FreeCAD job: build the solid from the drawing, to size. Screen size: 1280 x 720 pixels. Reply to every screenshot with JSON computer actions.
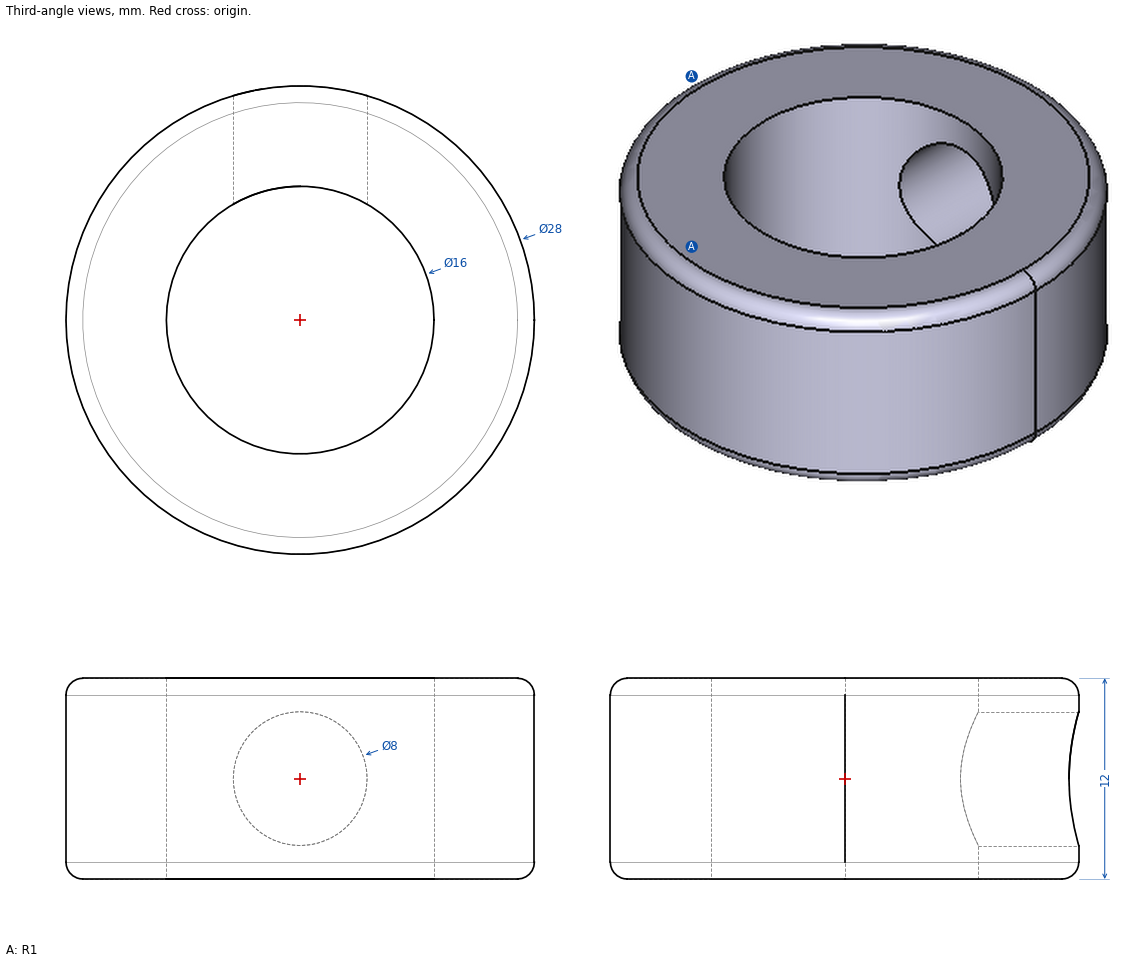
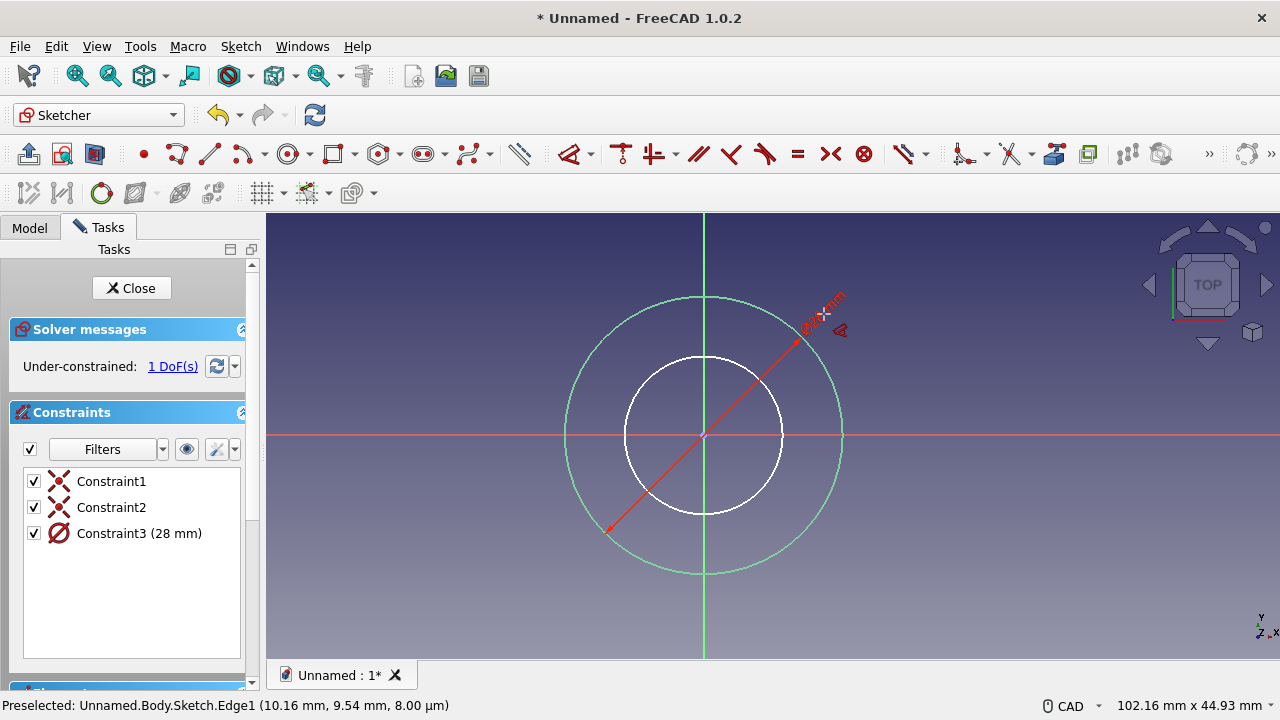
{"action": "left_click", "coordinate": [759, 379]}
{"action": "left_click", "coordinate": [781, 356]}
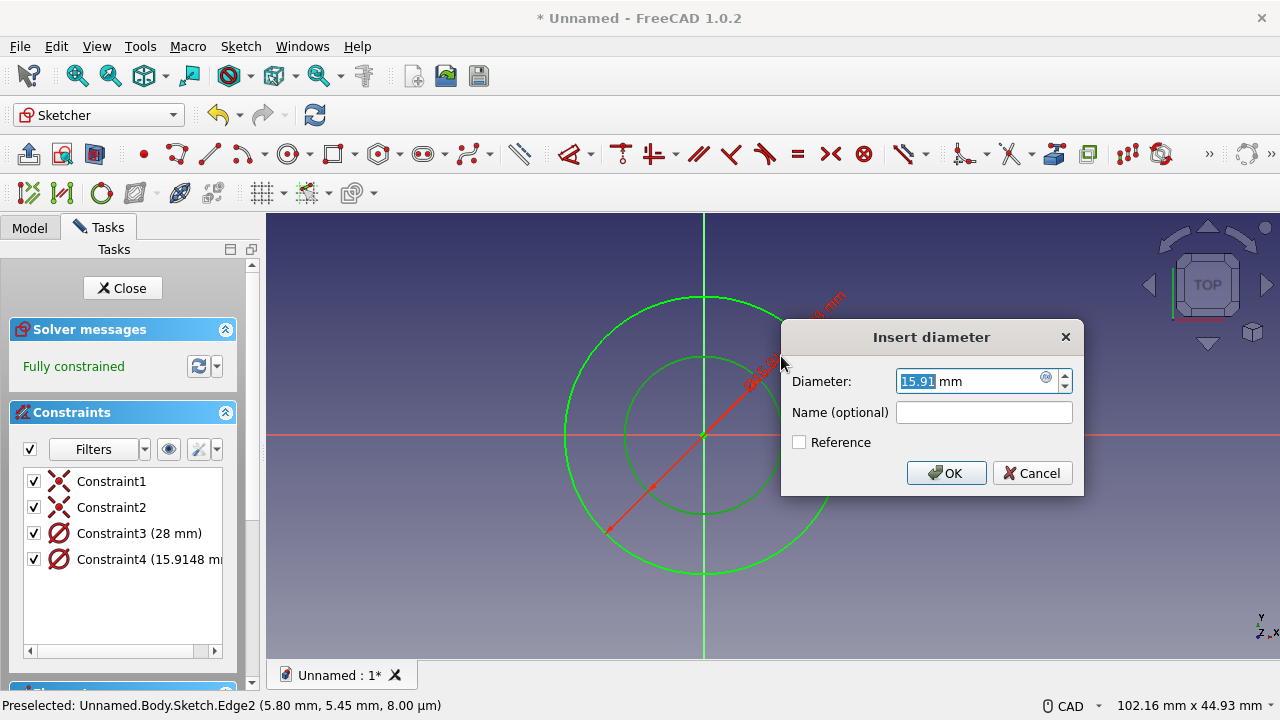
{"action": "type", "text": "16"}
{"action": "key", "text": "Return"}
{"action": "key", "text": "Escape"}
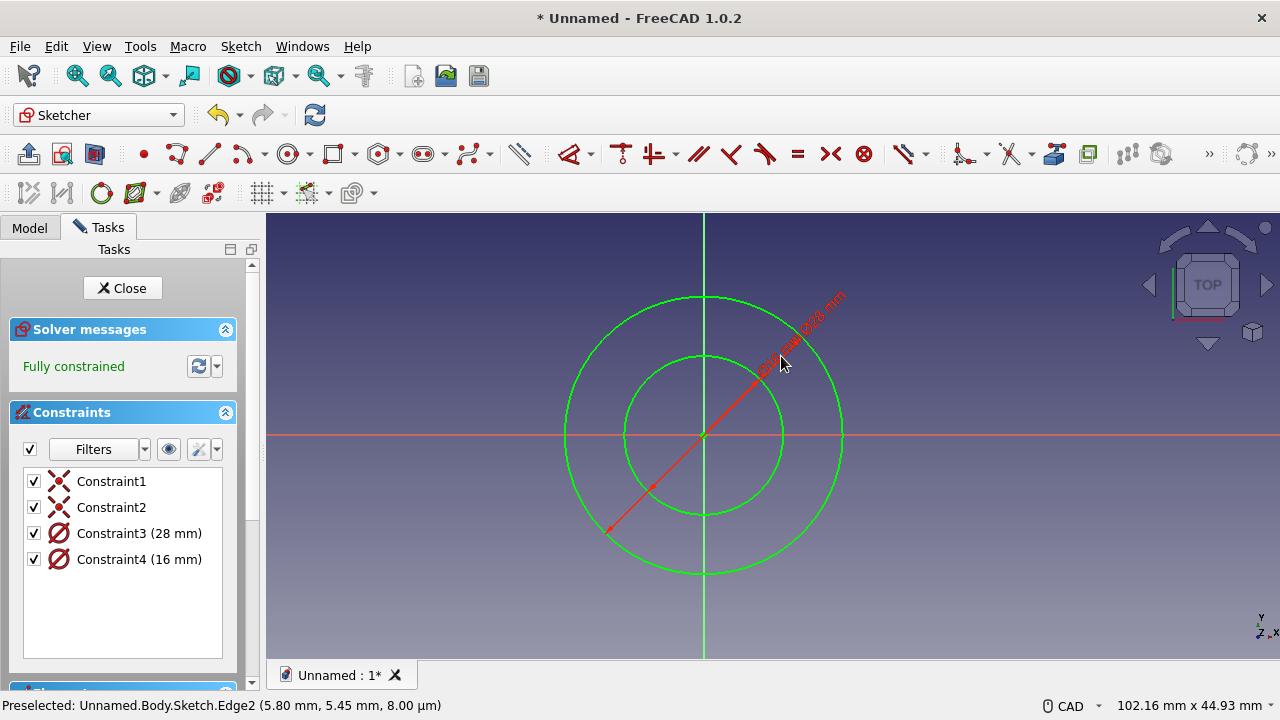
{"action": "left_click", "coordinate": [123, 288]}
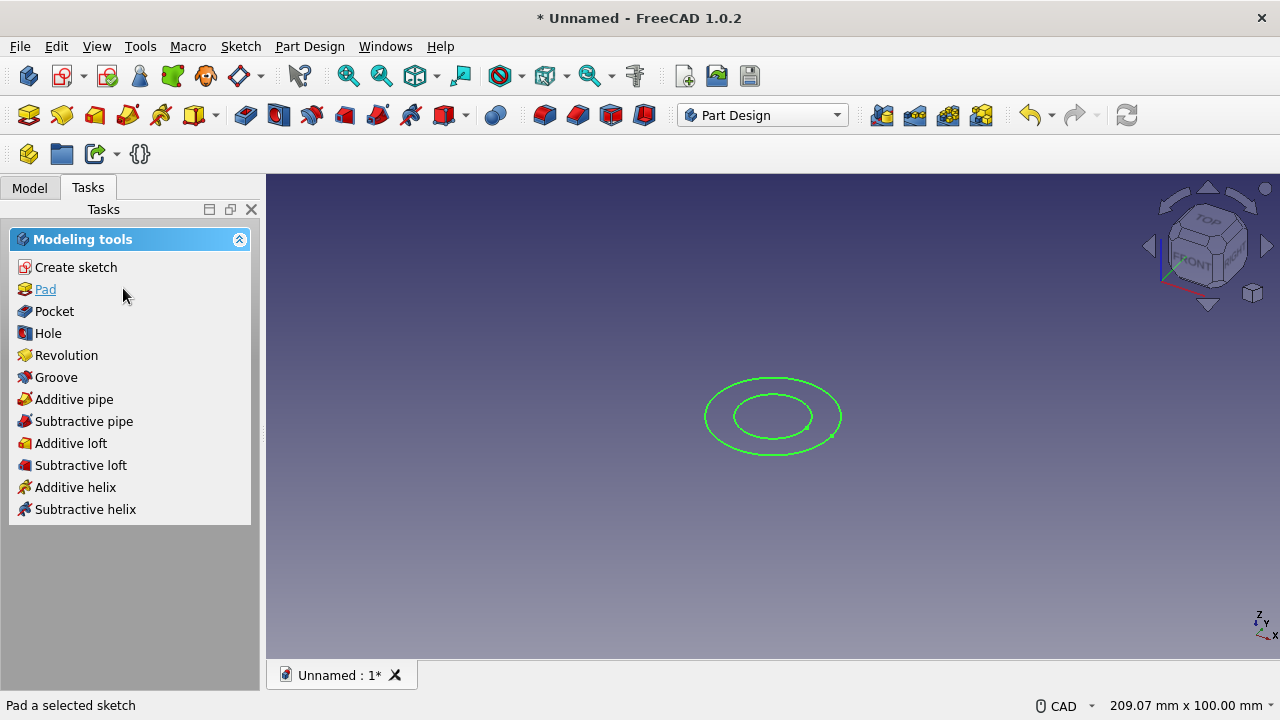
{"action": "left_click", "coordinate": [29, 116]}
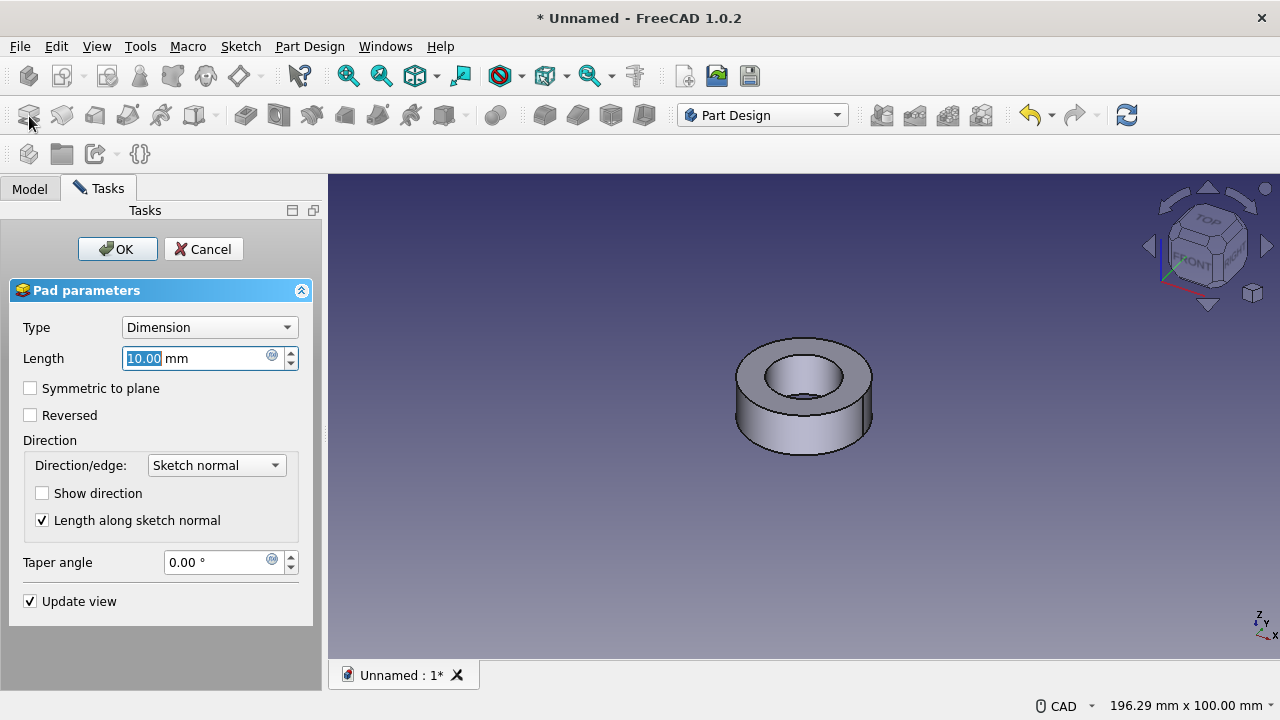
{"action": "type", "text": "12"}
{"action": "key", "text": "Tab"}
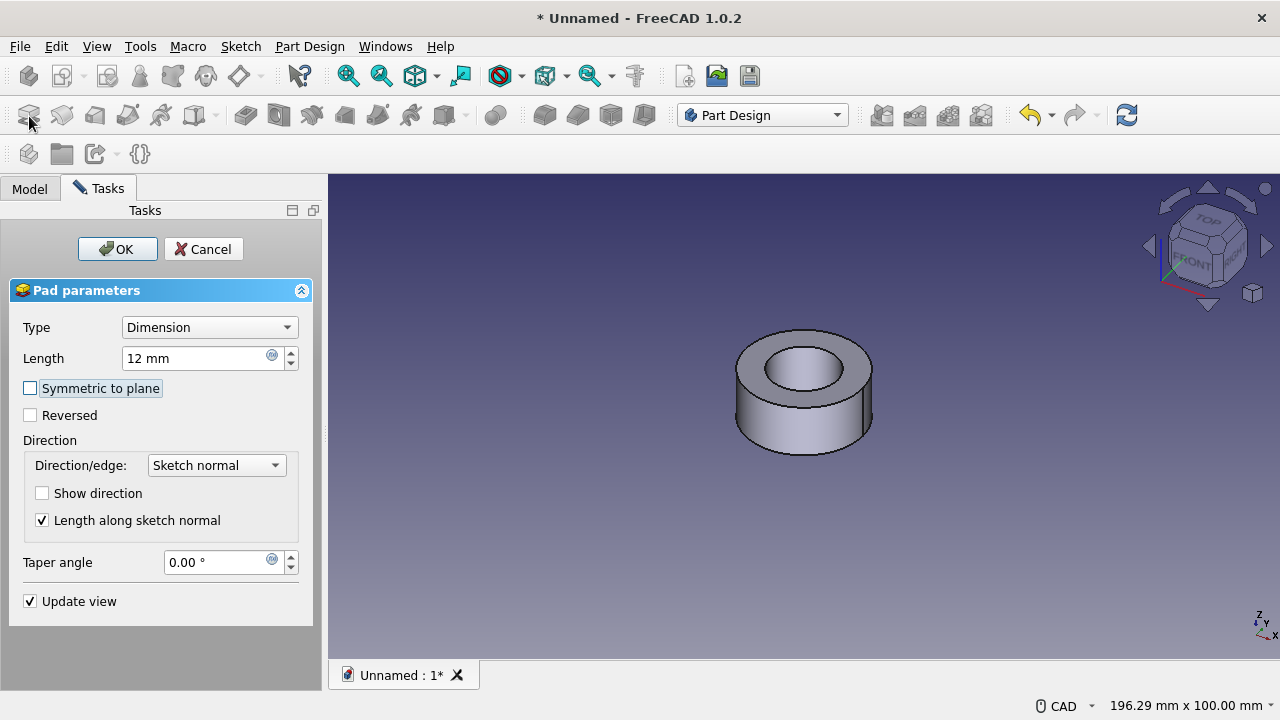
{"action": "left_click", "coordinate": [31, 388]}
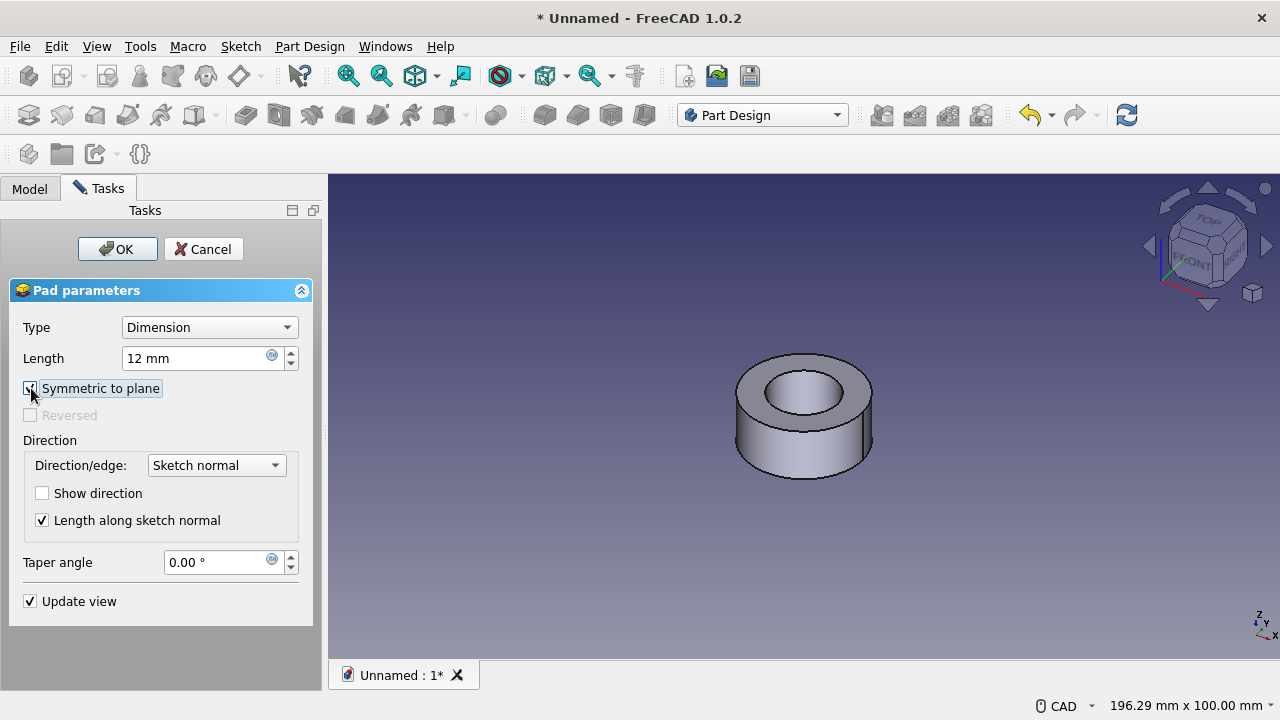
{"action": "left_click", "coordinate": [118, 249]}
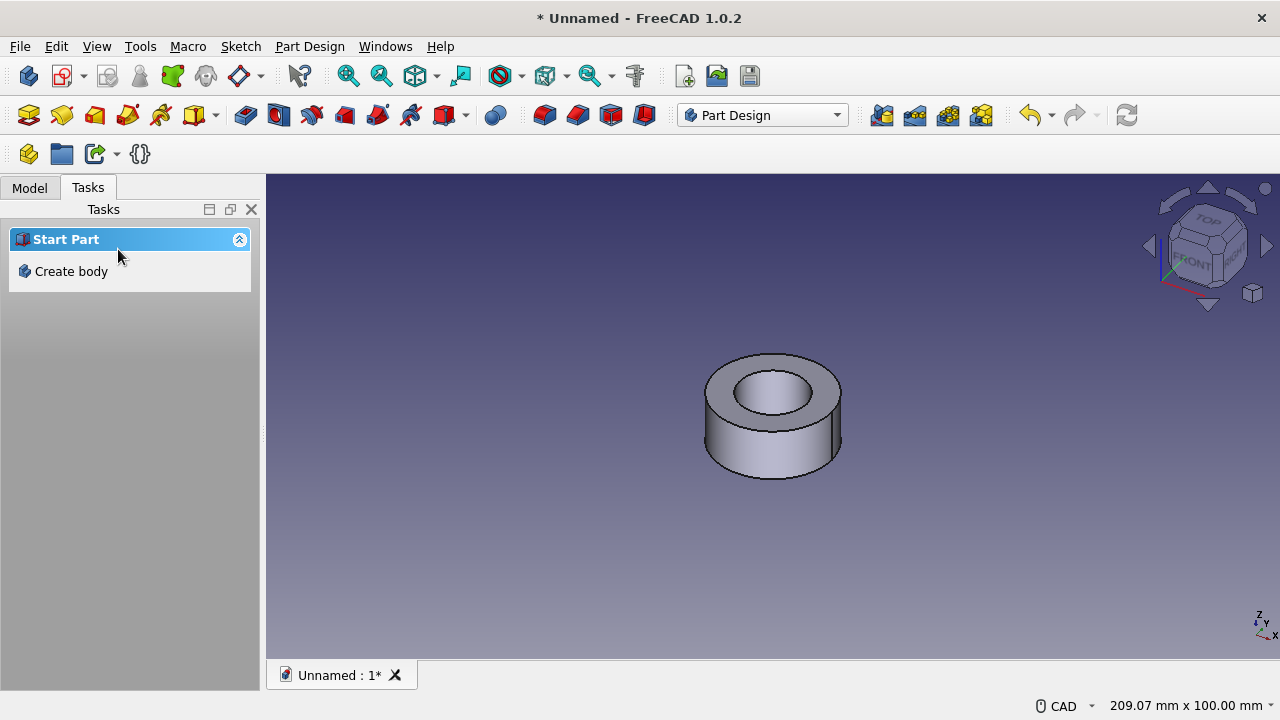
{"action": "key", "text": "v f"}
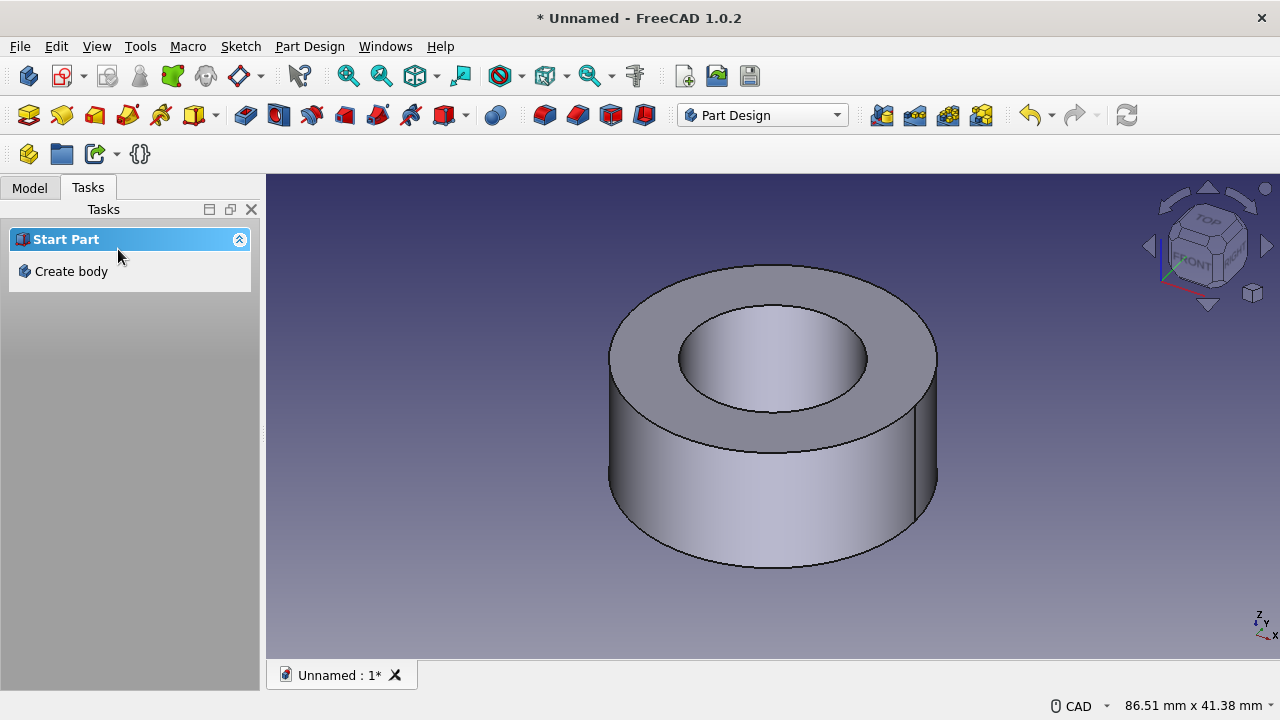
{"action": "left_click", "coordinate": [610, 368]}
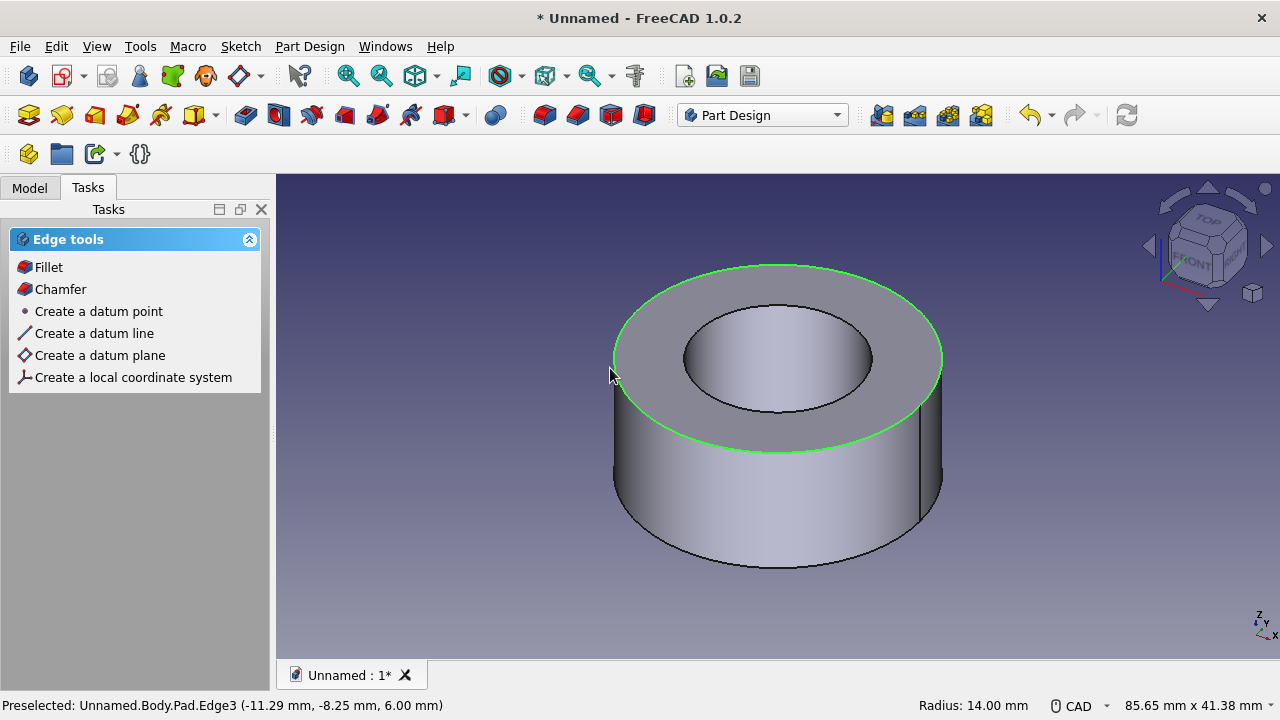
{"action": "key", "text": "0"}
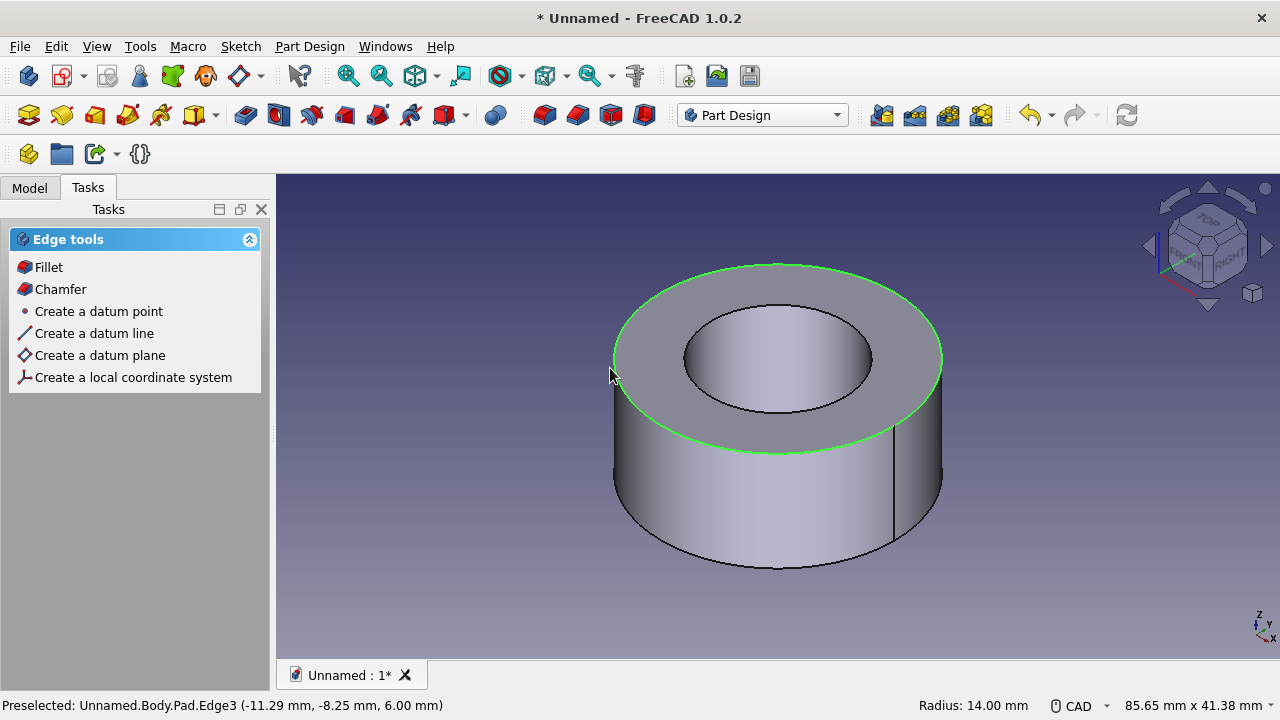
{"action": "key", "text": "2"}